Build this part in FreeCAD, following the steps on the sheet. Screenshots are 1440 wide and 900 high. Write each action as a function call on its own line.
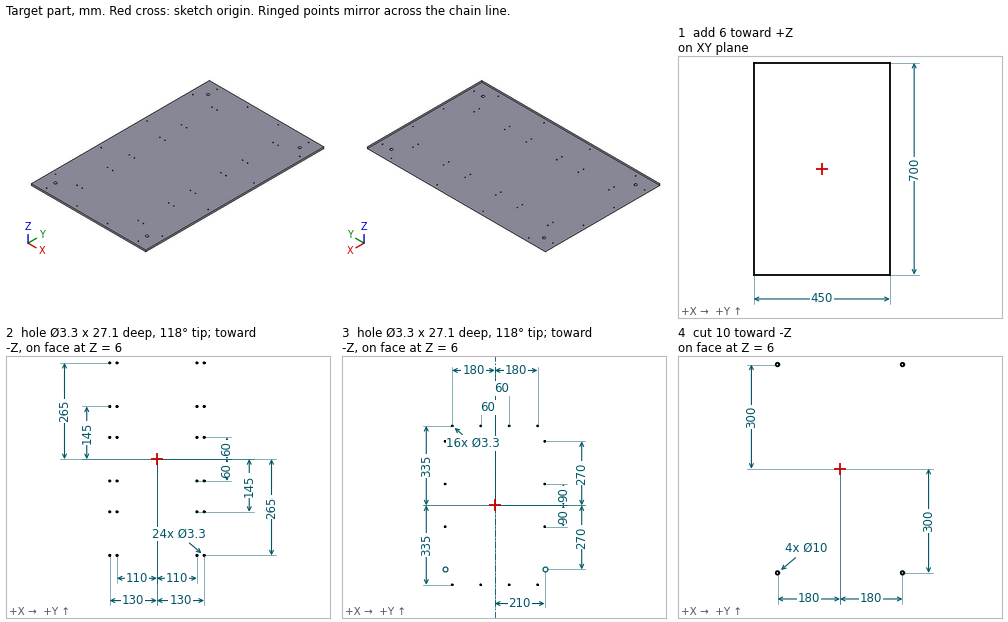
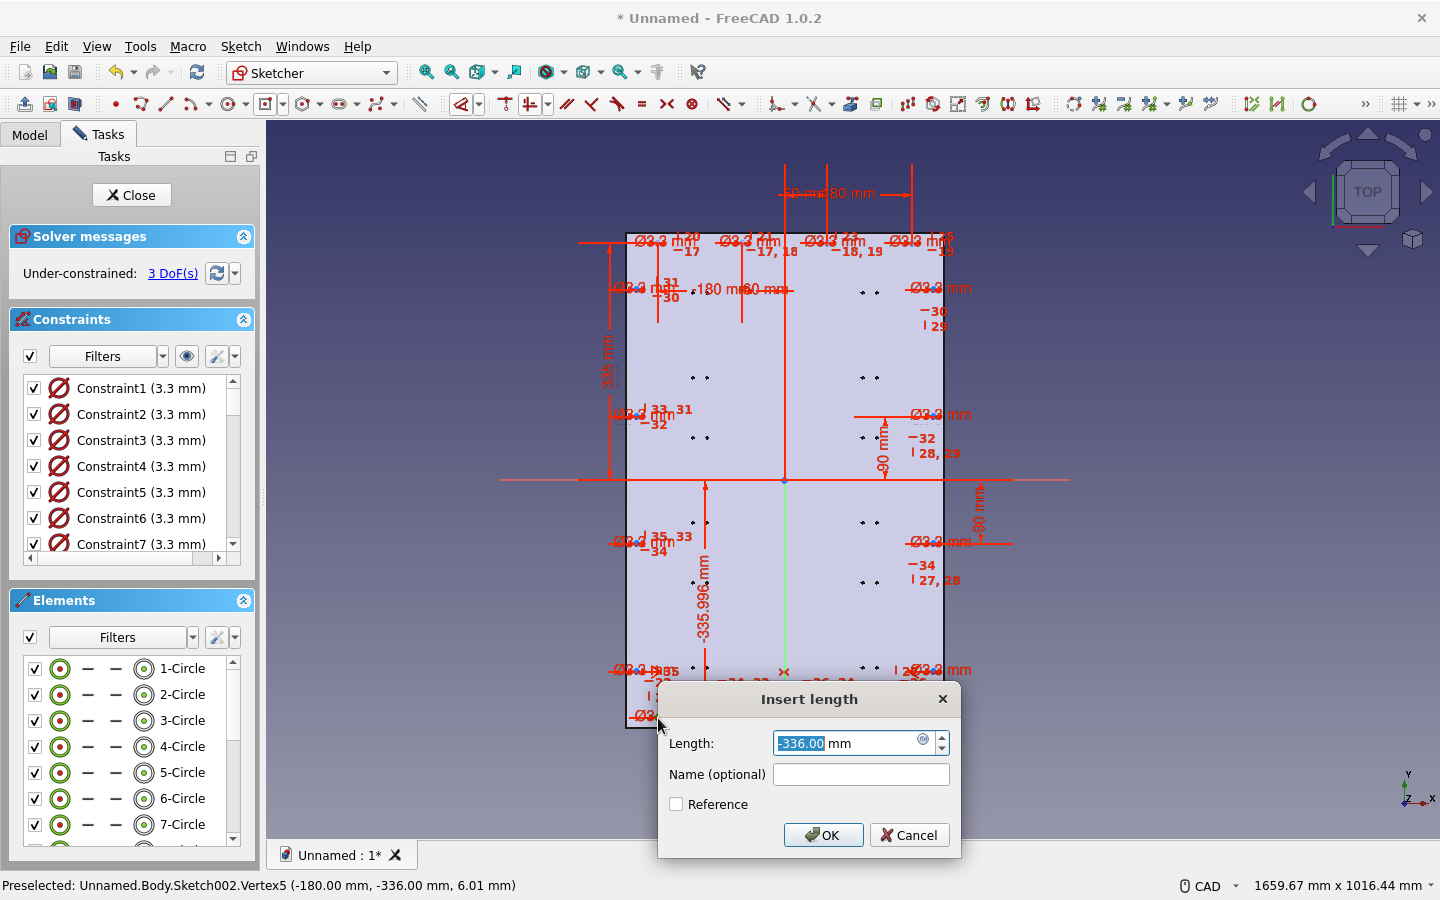
text(-335)
key(Return)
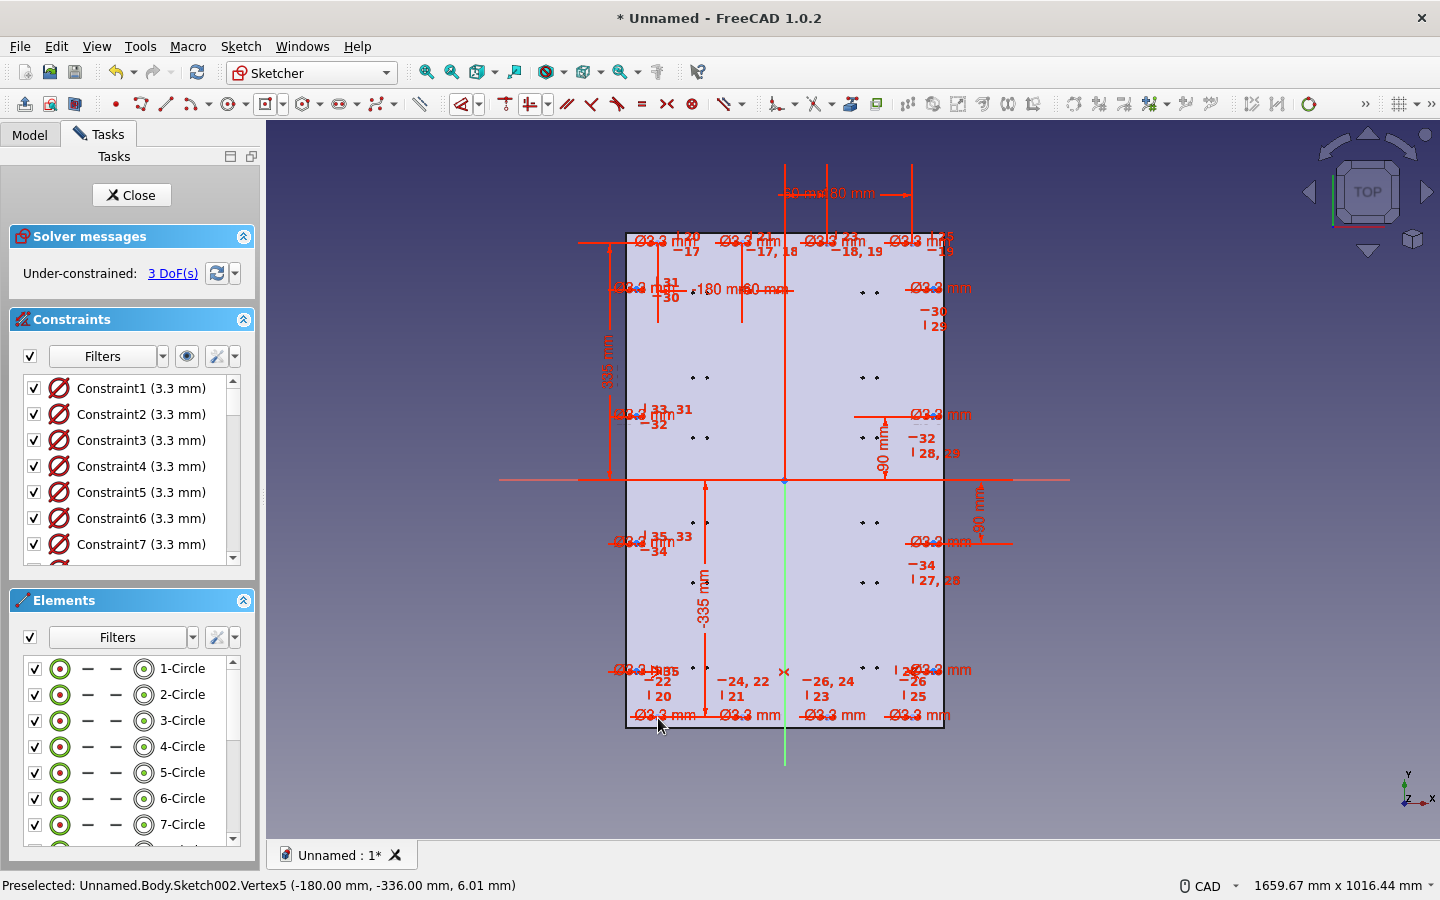
click(933, 672)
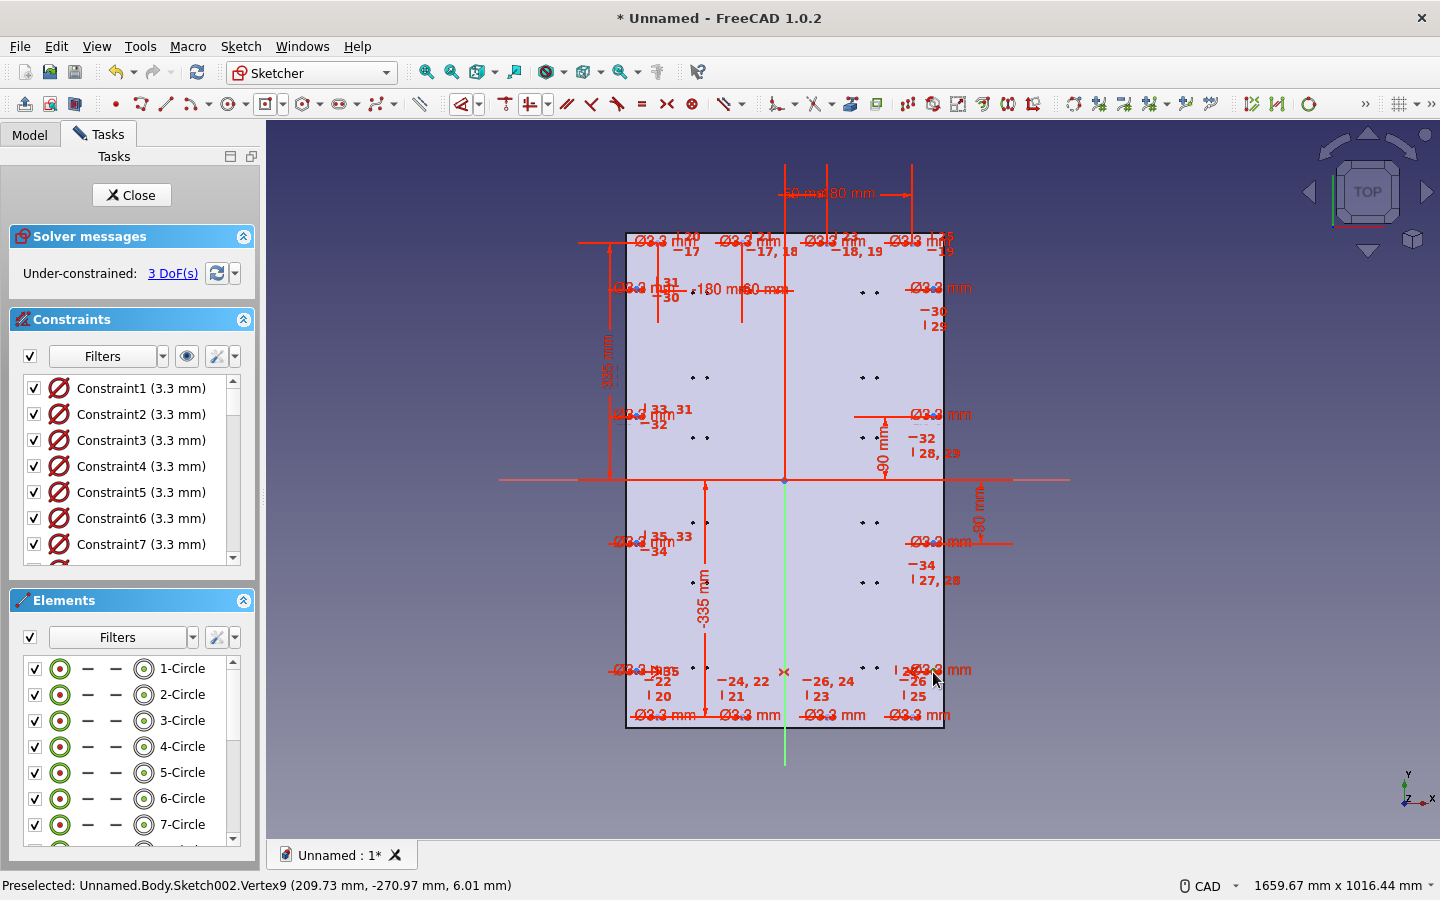
key(l)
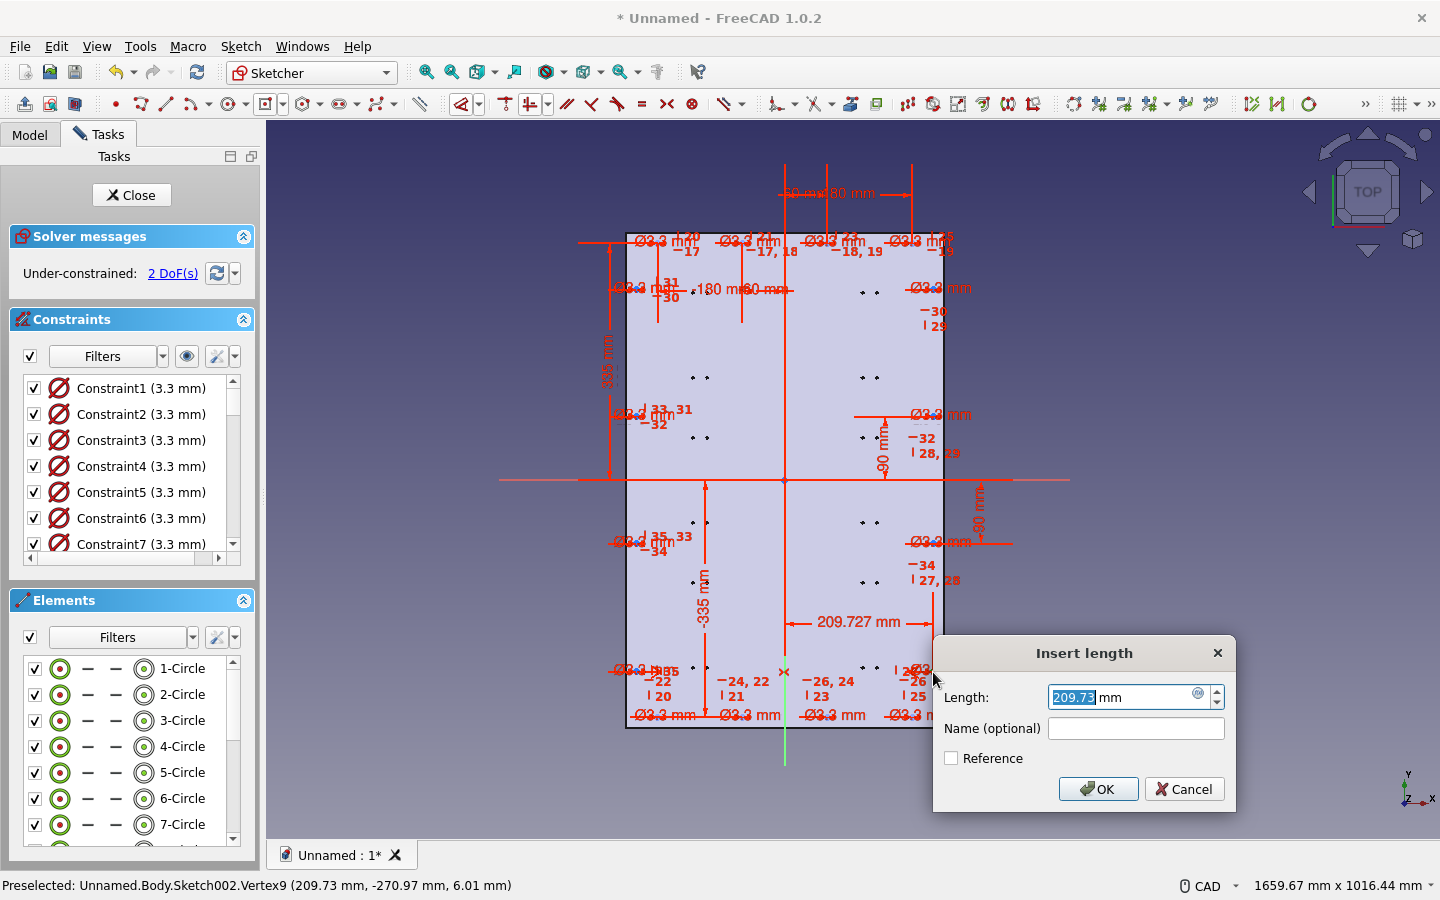
text(210)
key(Return)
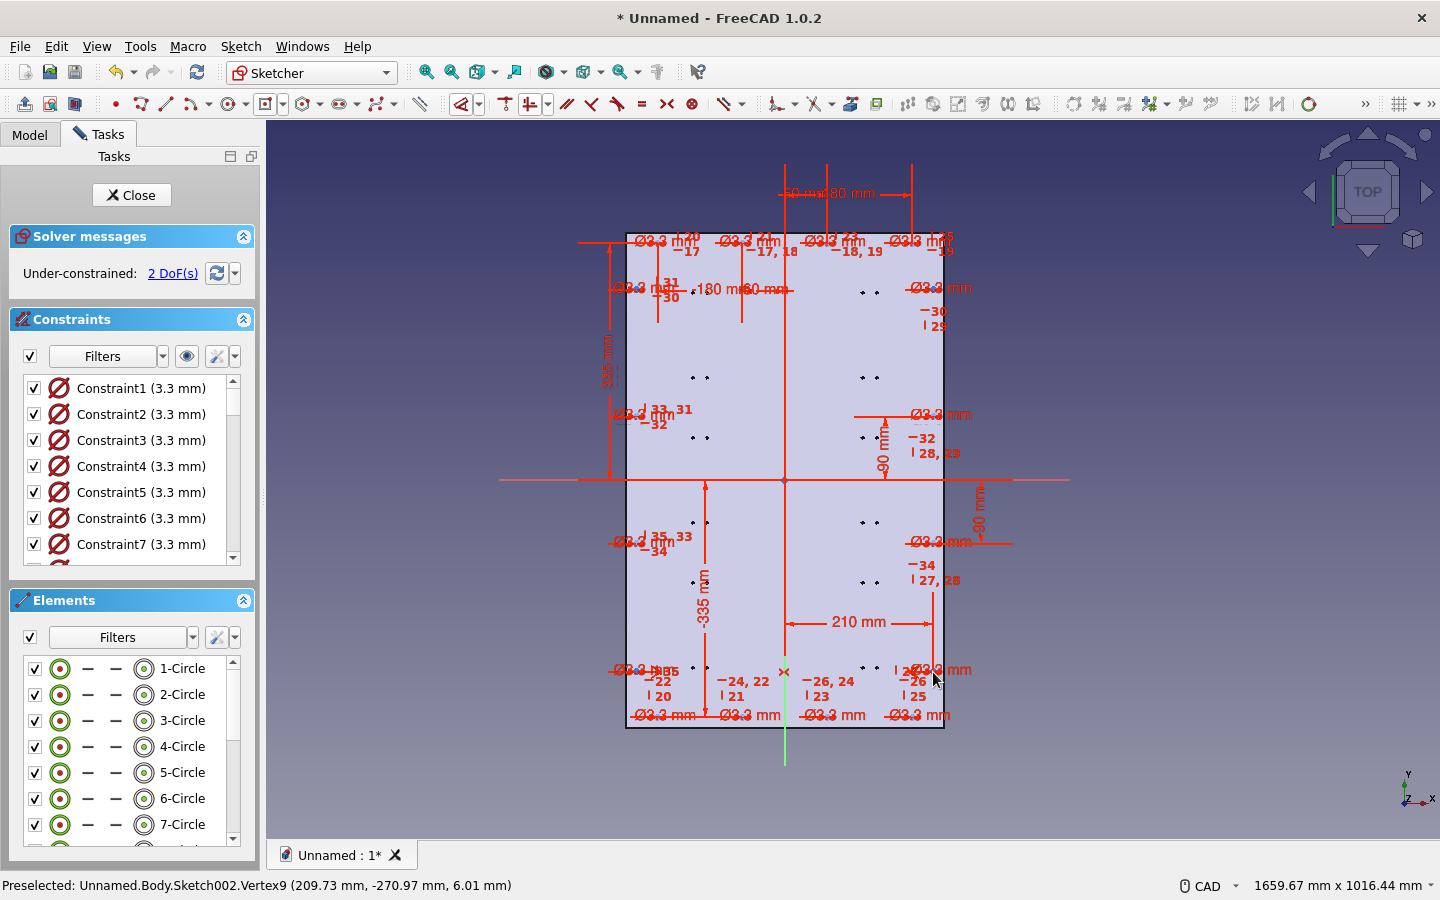
click(933, 672)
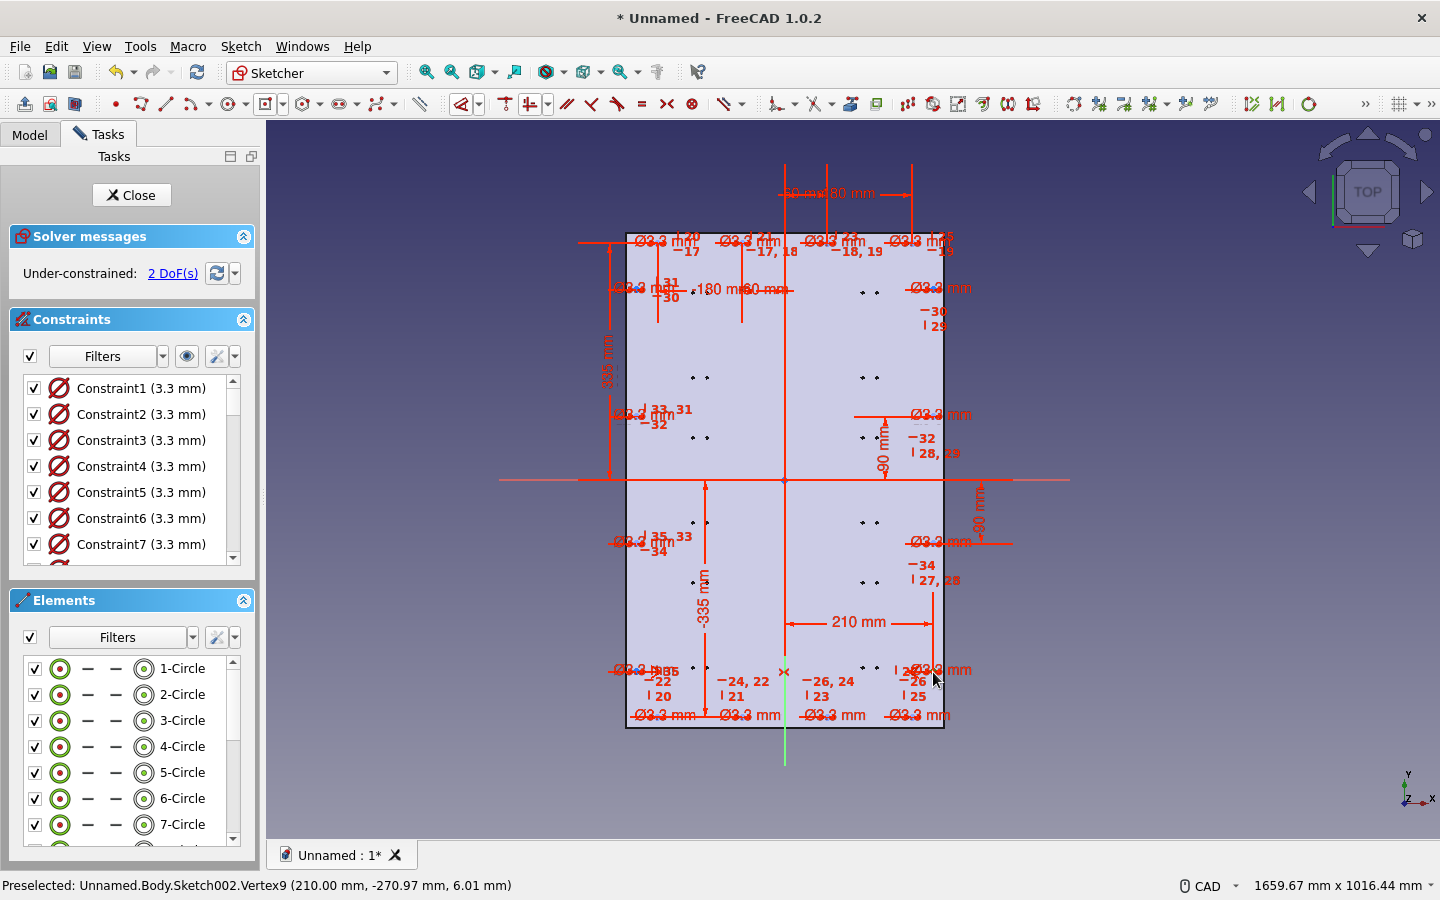
click(478, 104)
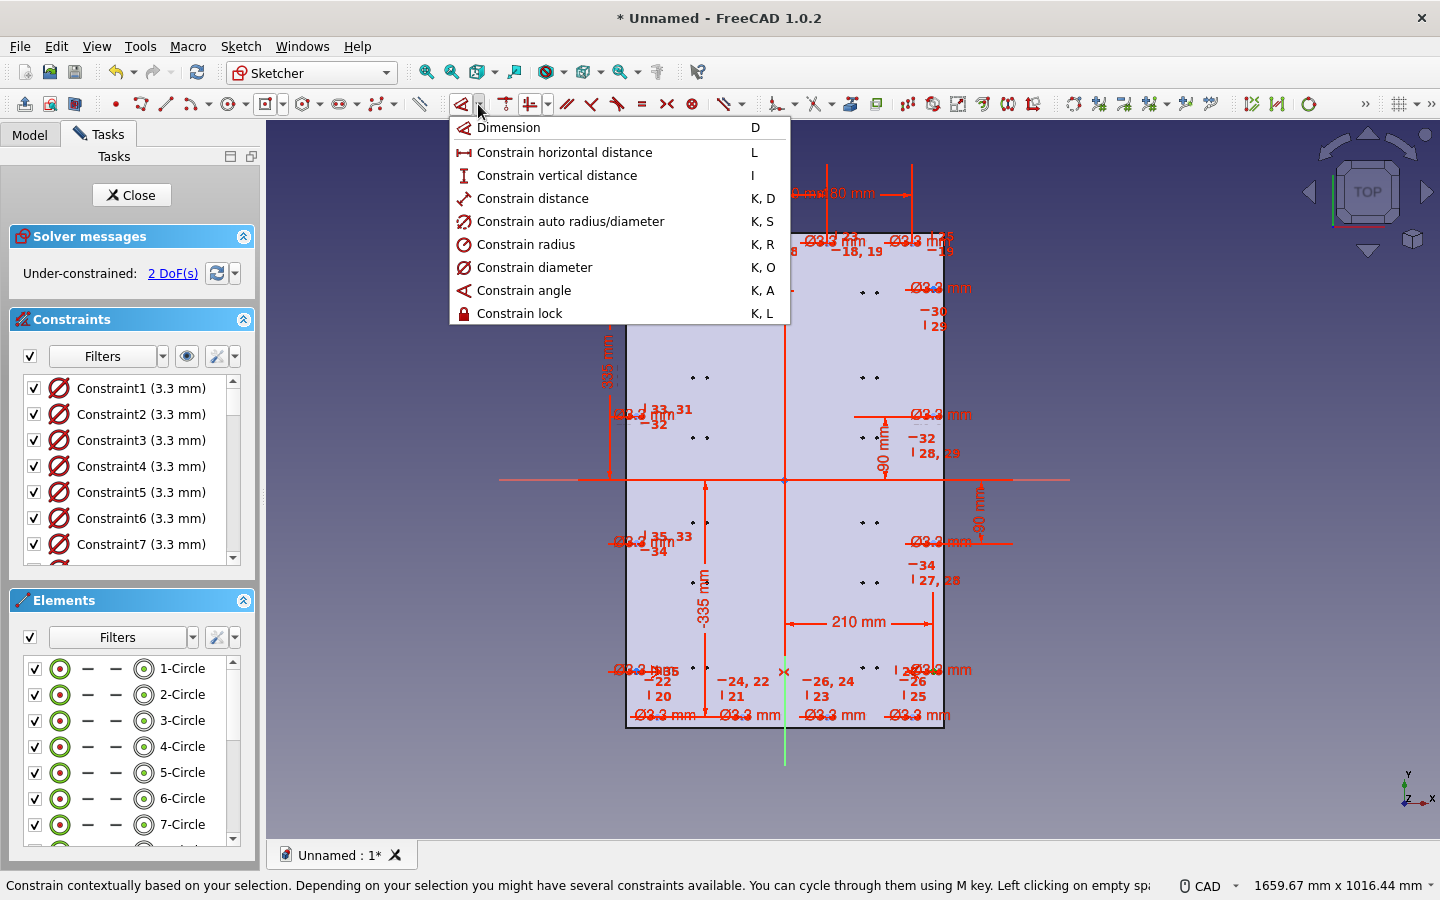
click(620, 176)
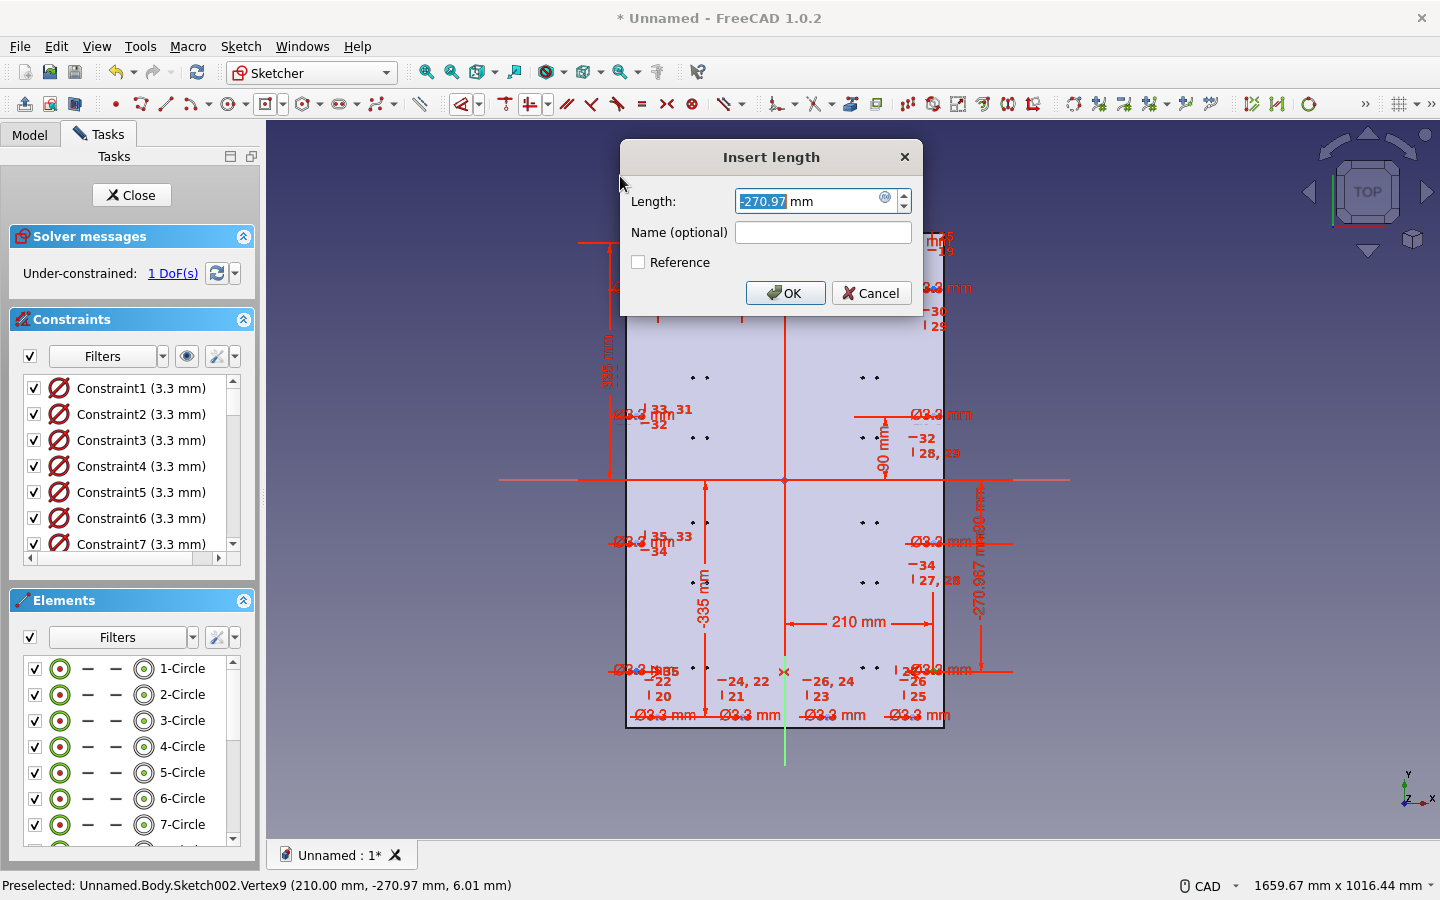
text(-270)
key(Return)